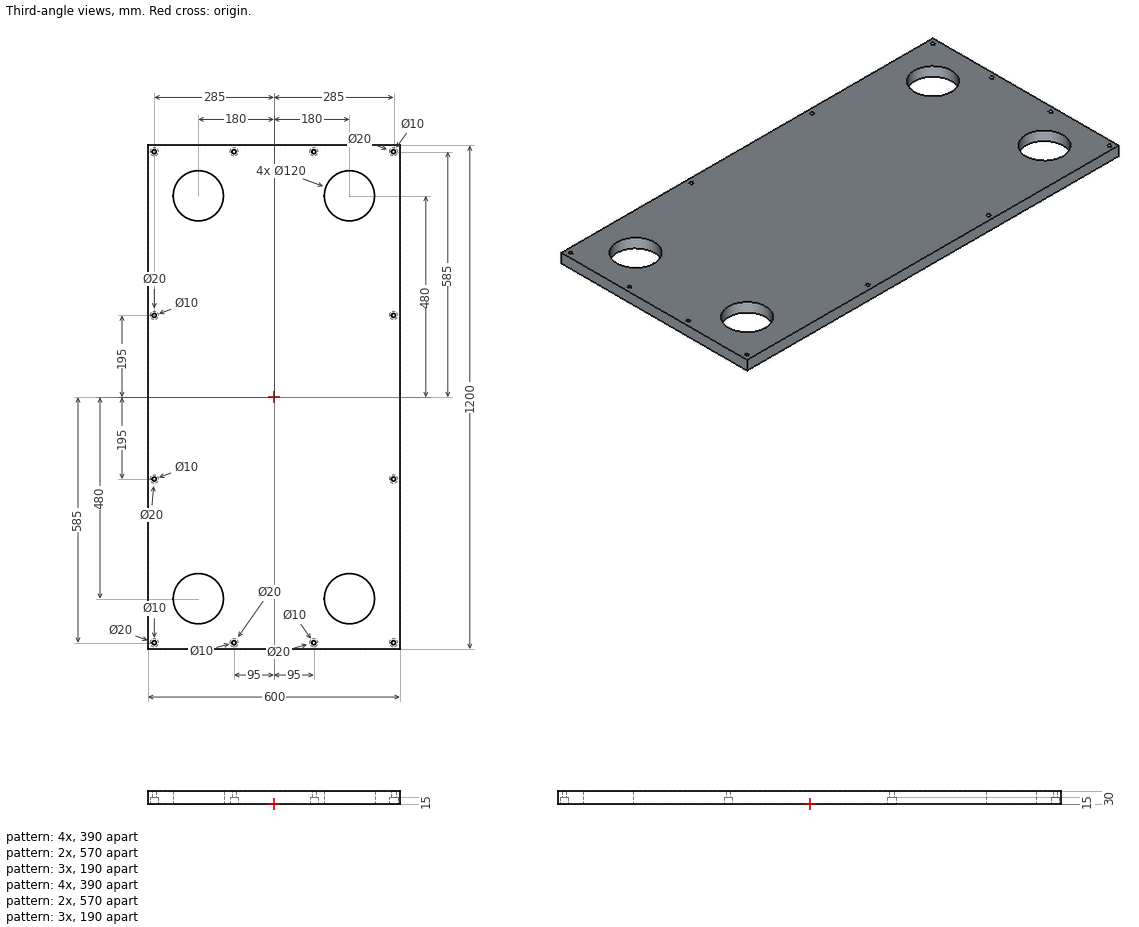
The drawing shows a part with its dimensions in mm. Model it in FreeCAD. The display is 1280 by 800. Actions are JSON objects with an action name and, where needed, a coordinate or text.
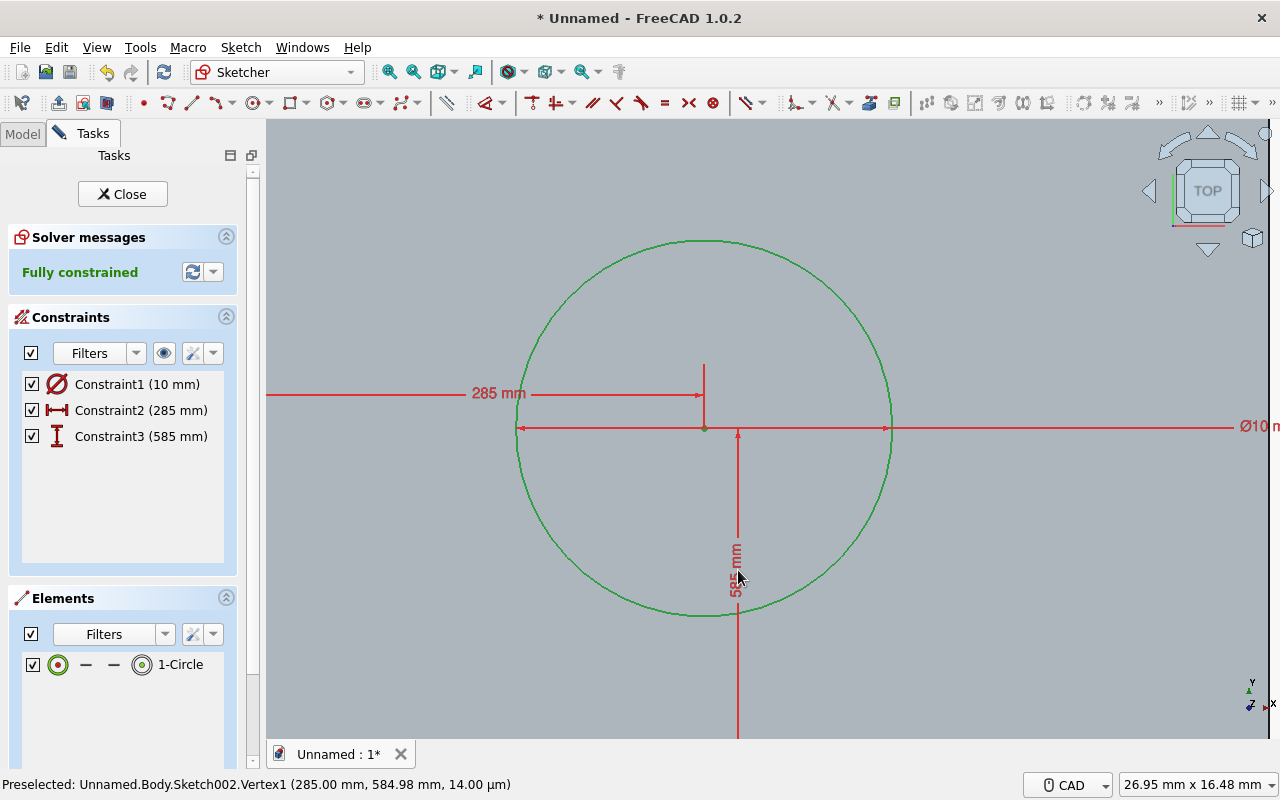
{"action": "left_click", "coordinate": [123, 194]}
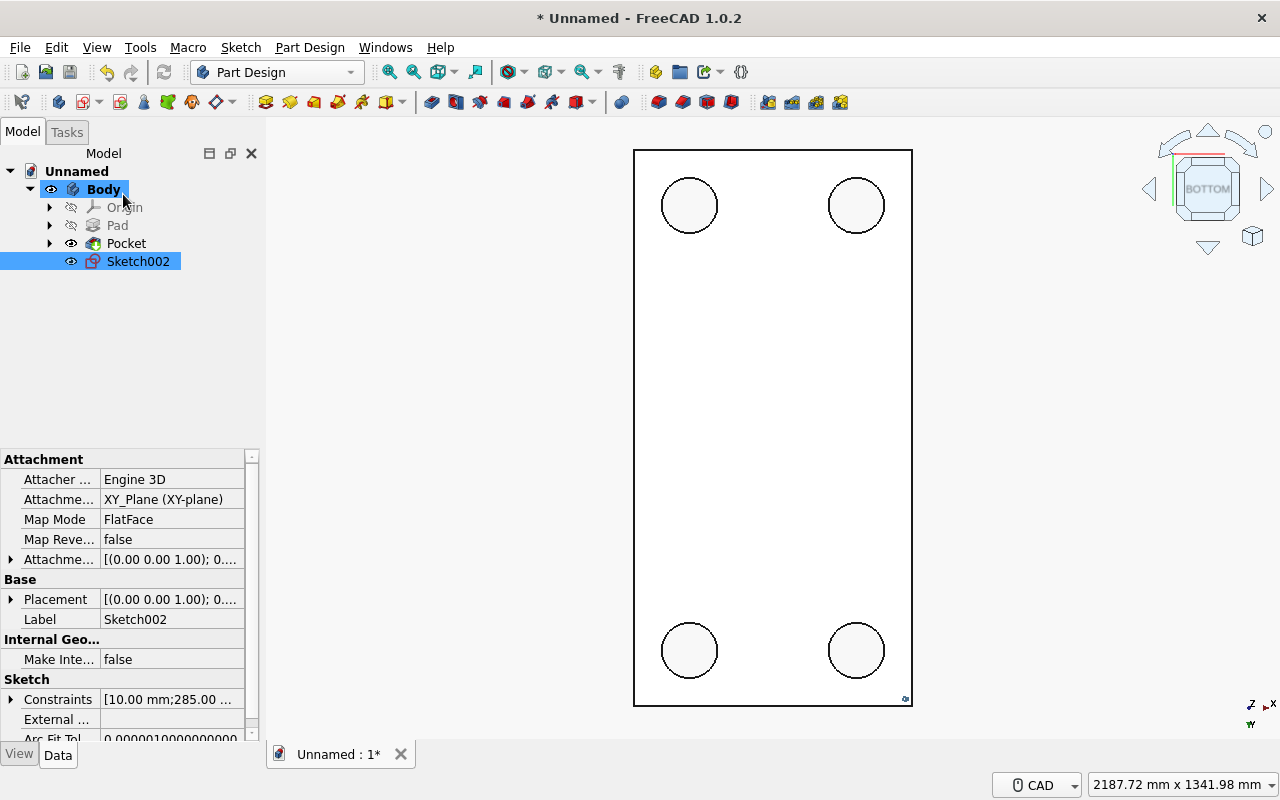
{"action": "left_click", "coordinate": [432, 102]}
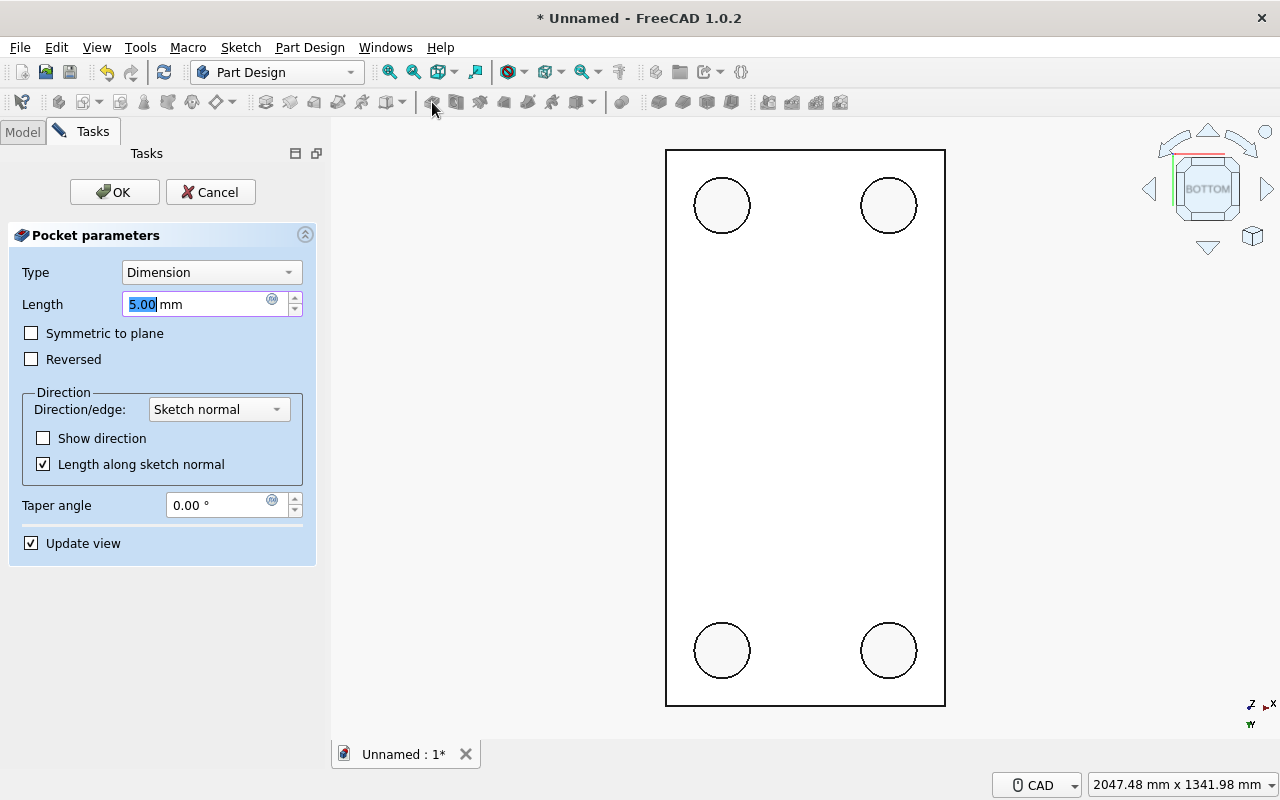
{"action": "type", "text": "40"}
{"action": "key", "text": "Tab"}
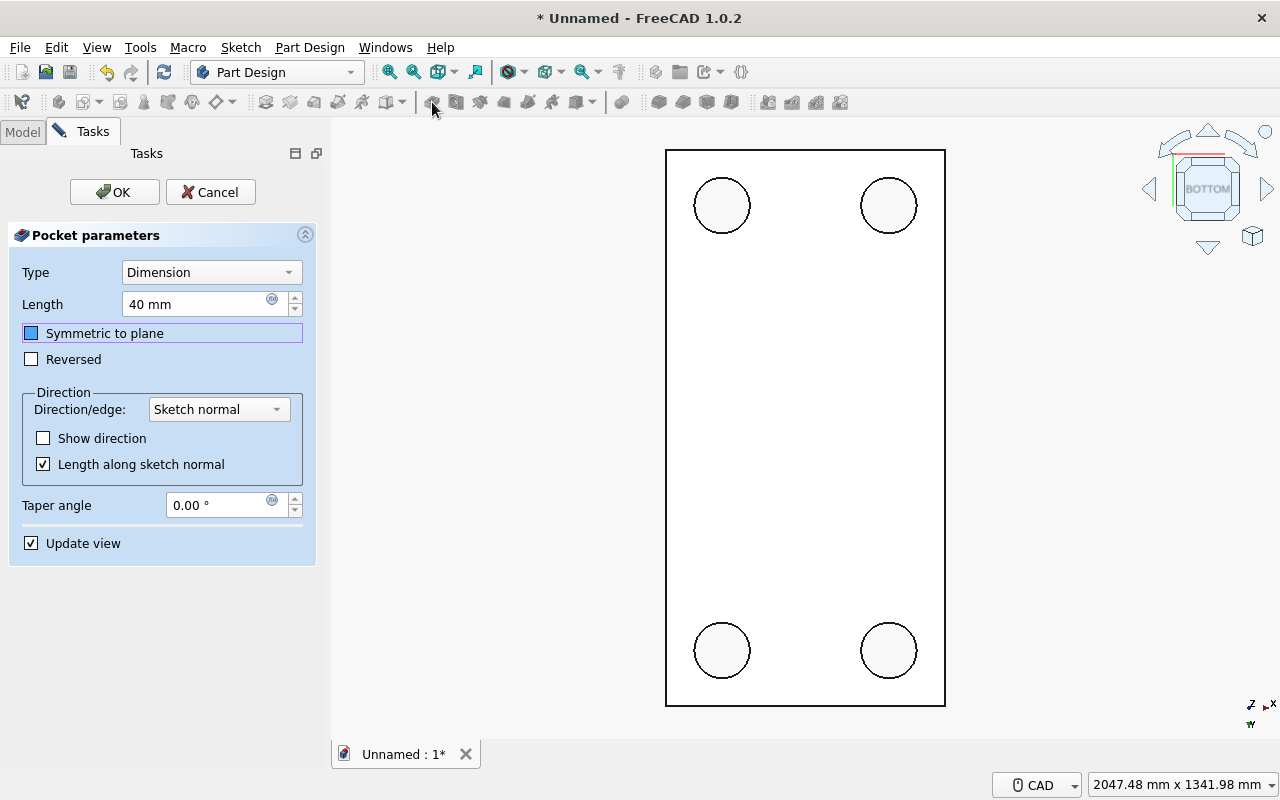
{"action": "left_click", "coordinate": [30, 359]}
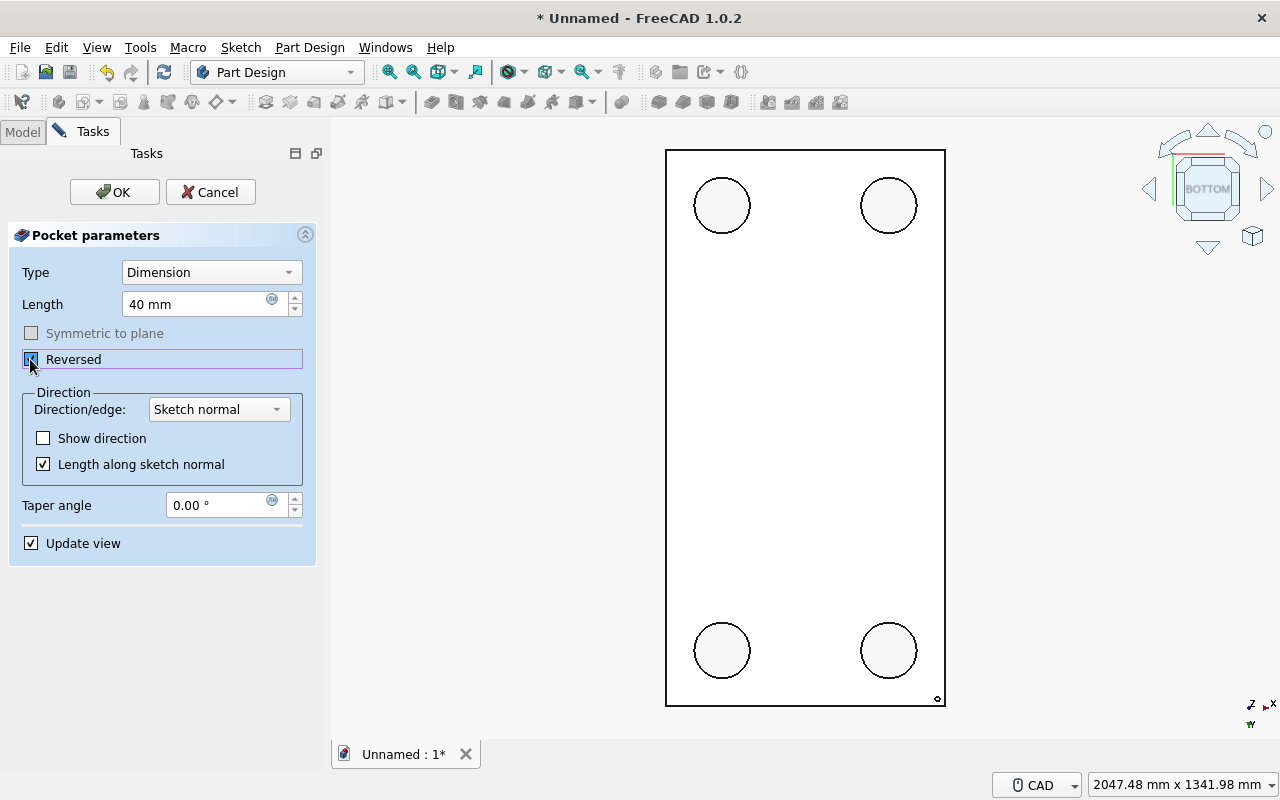
{"action": "left_click", "coordinate": [115, 192]}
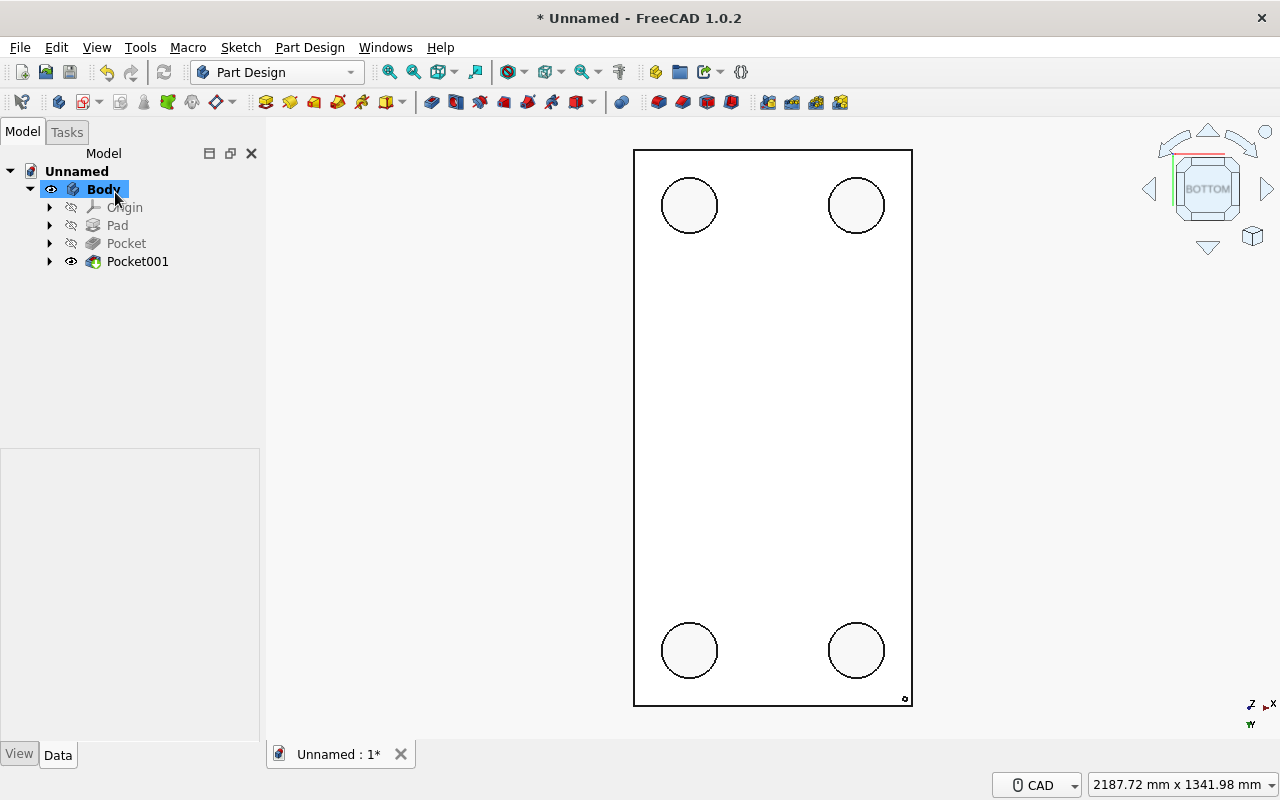
{"action": "left_click", "coordinate": [116, 261]}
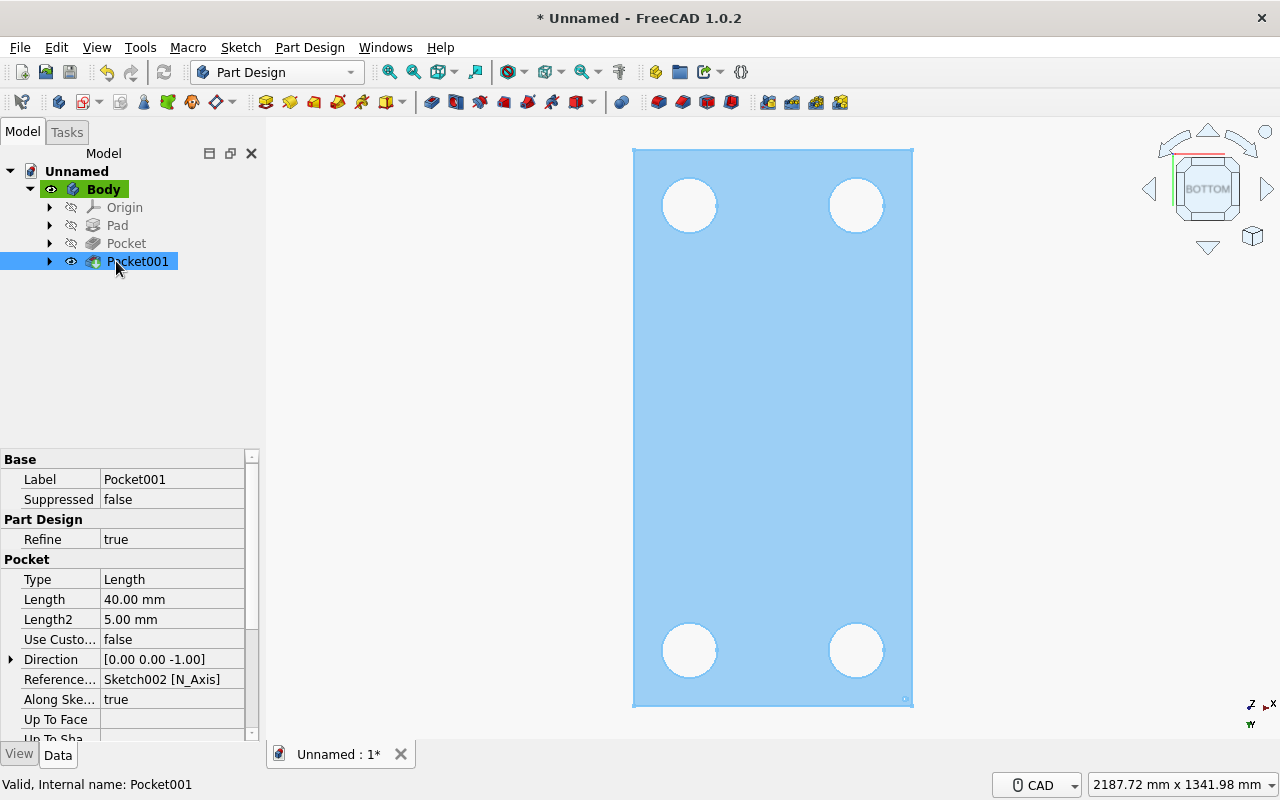
{"action": "left_click", "coordinate": [792, 102]}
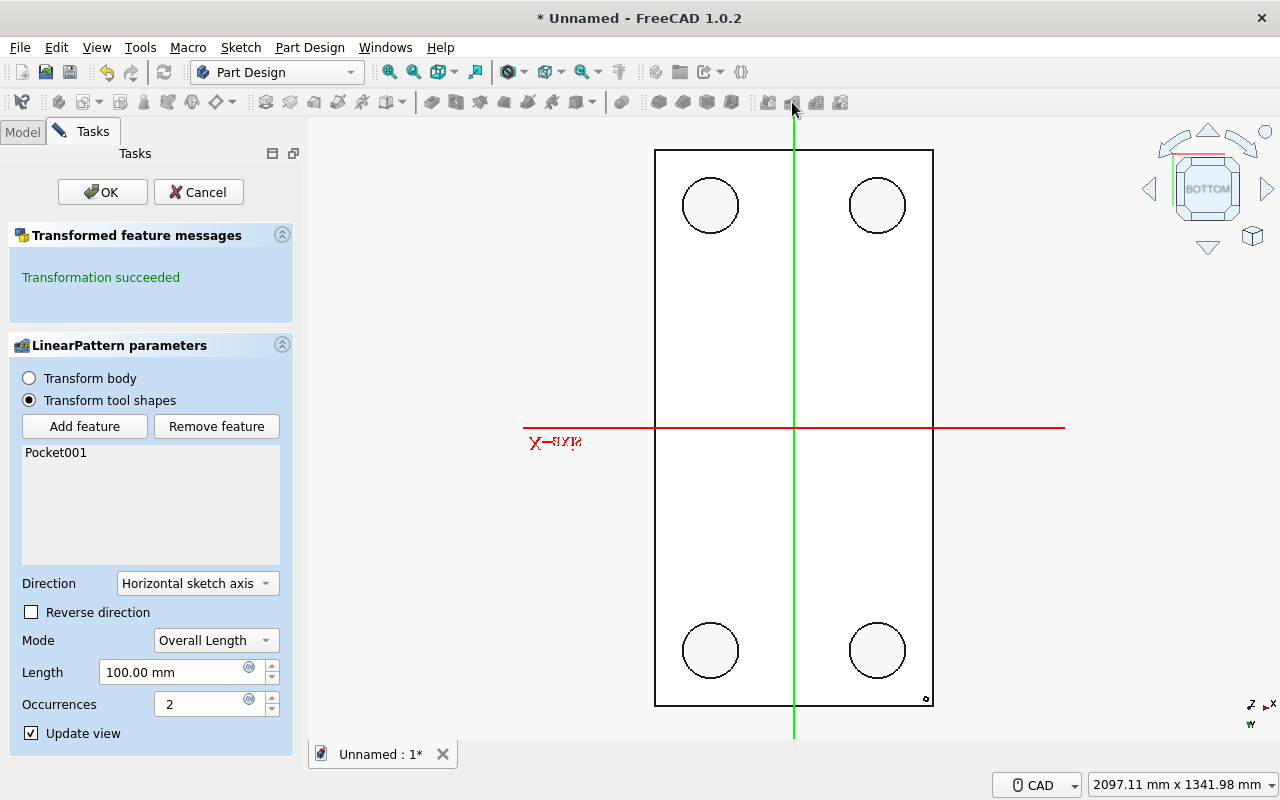
{"action": "left_click", "coordinate": [198, 584]}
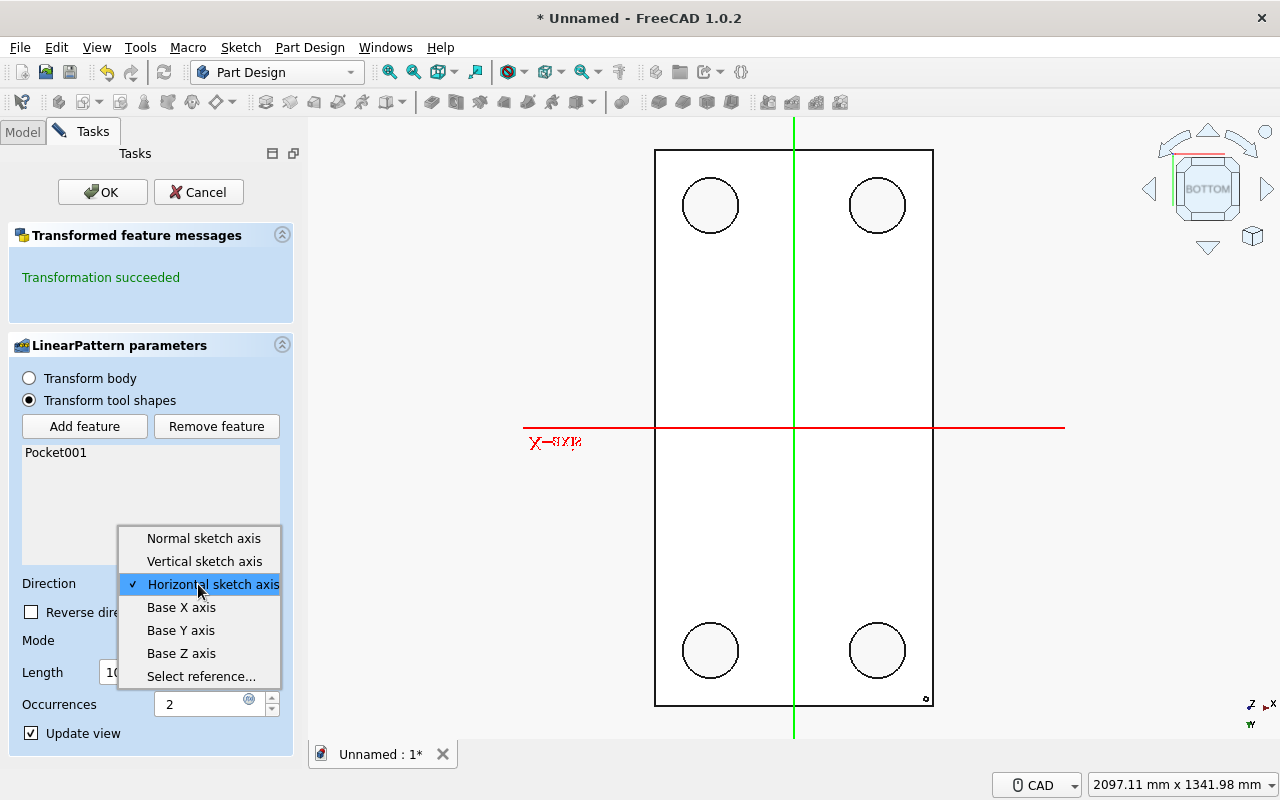
{"action": "left_click", "coordinate": [198, 630]}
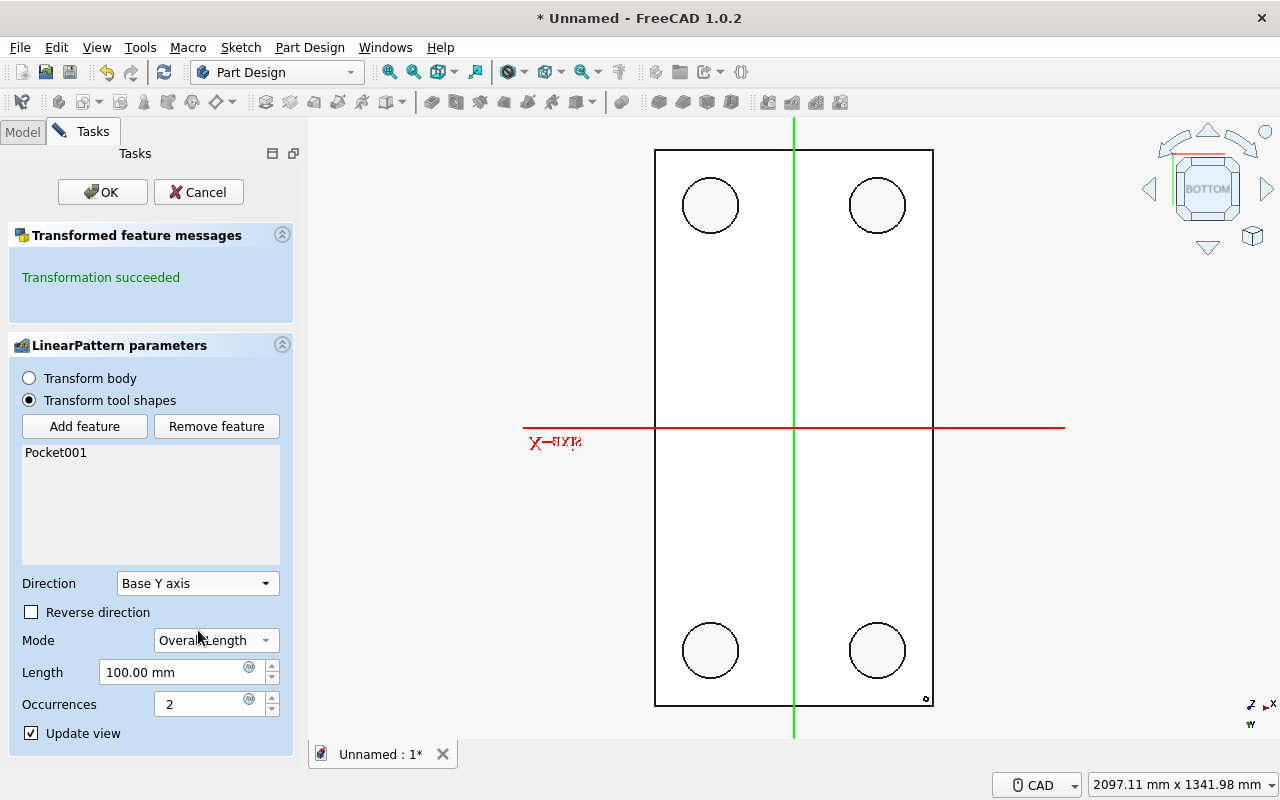
{"action": "left_click", "coordinate": [217, 640]}